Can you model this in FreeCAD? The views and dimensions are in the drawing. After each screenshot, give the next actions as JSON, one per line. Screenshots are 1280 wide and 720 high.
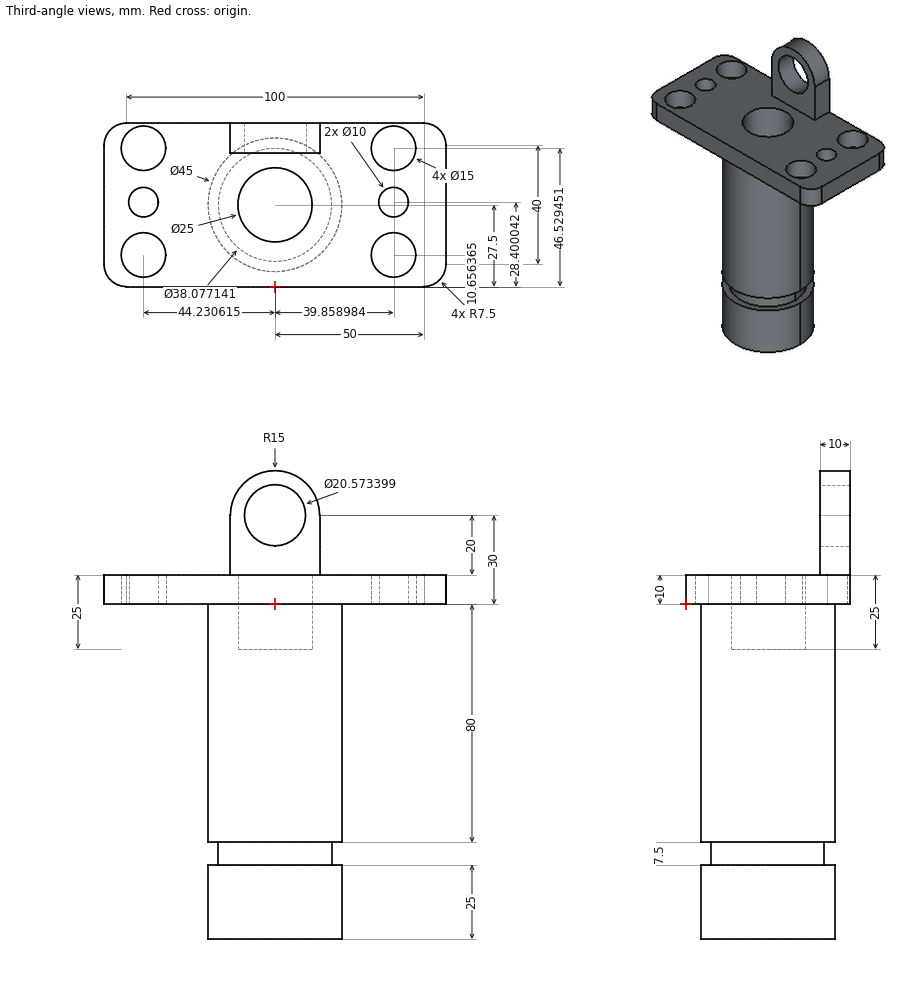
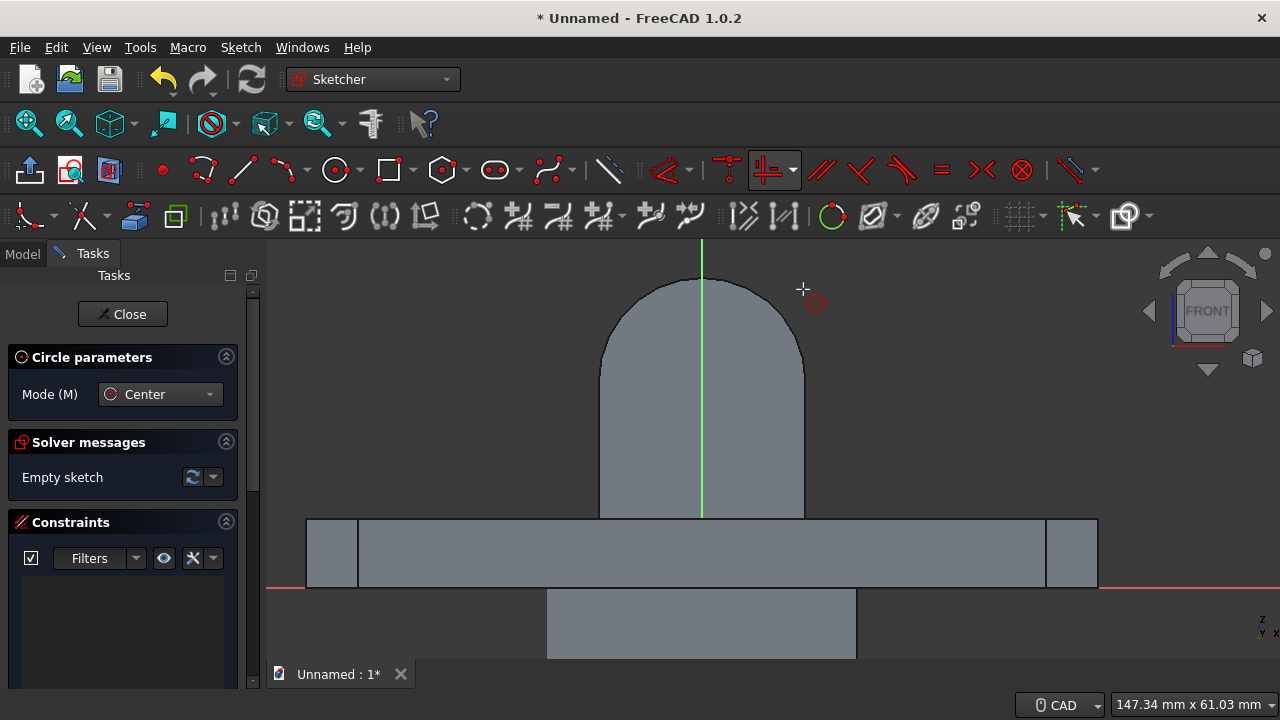
{"action": "left_click", "coordinate": [702, 381]}
{"action": "left_click", "coordinate": [752, 331]}
{"action": "key", "text": "Escape"}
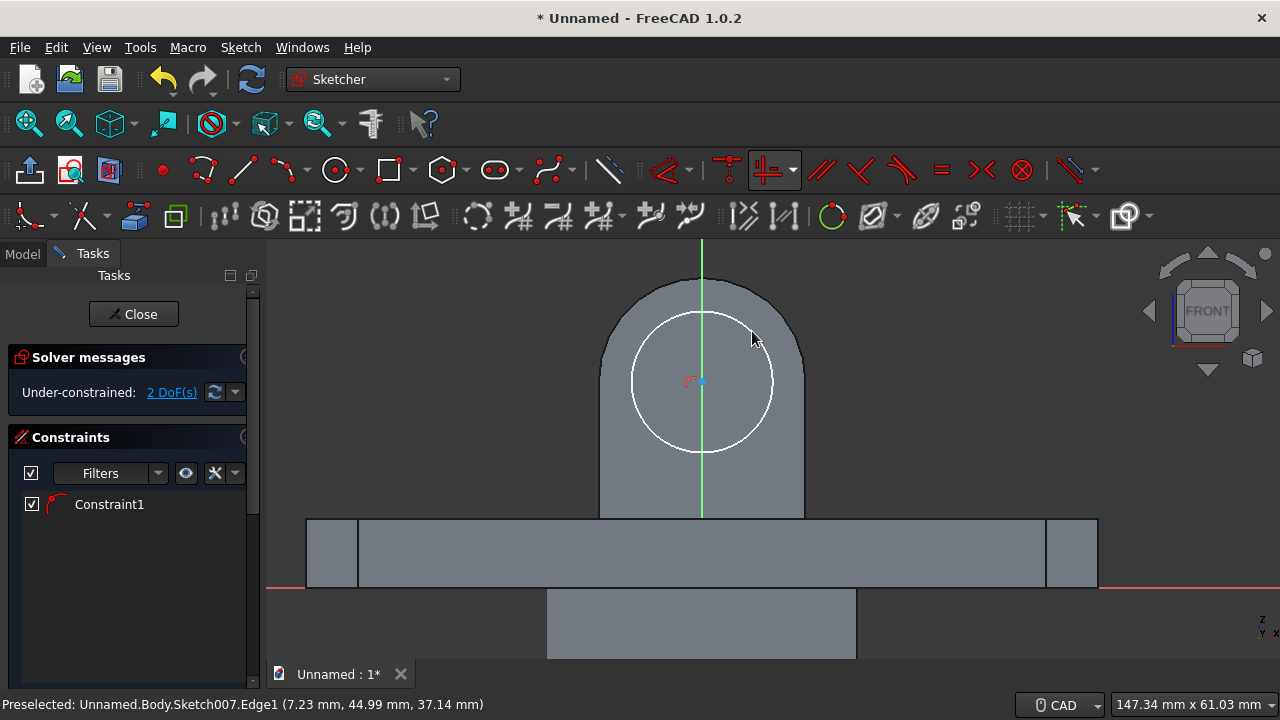
{"action": "left_click", "coordinate": [664, 170]}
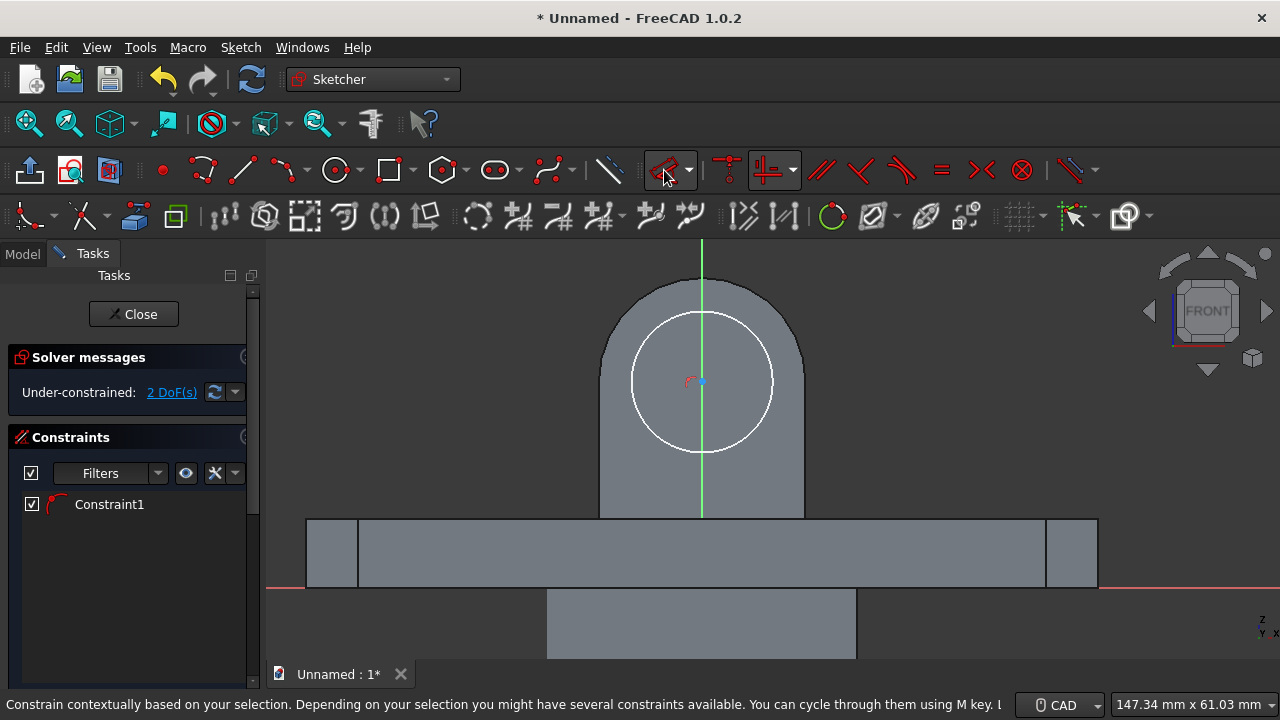
{"action": "left_click", "coordinate": [752, 332]}
{"action": "left_click", "coordinate": [775, 309]}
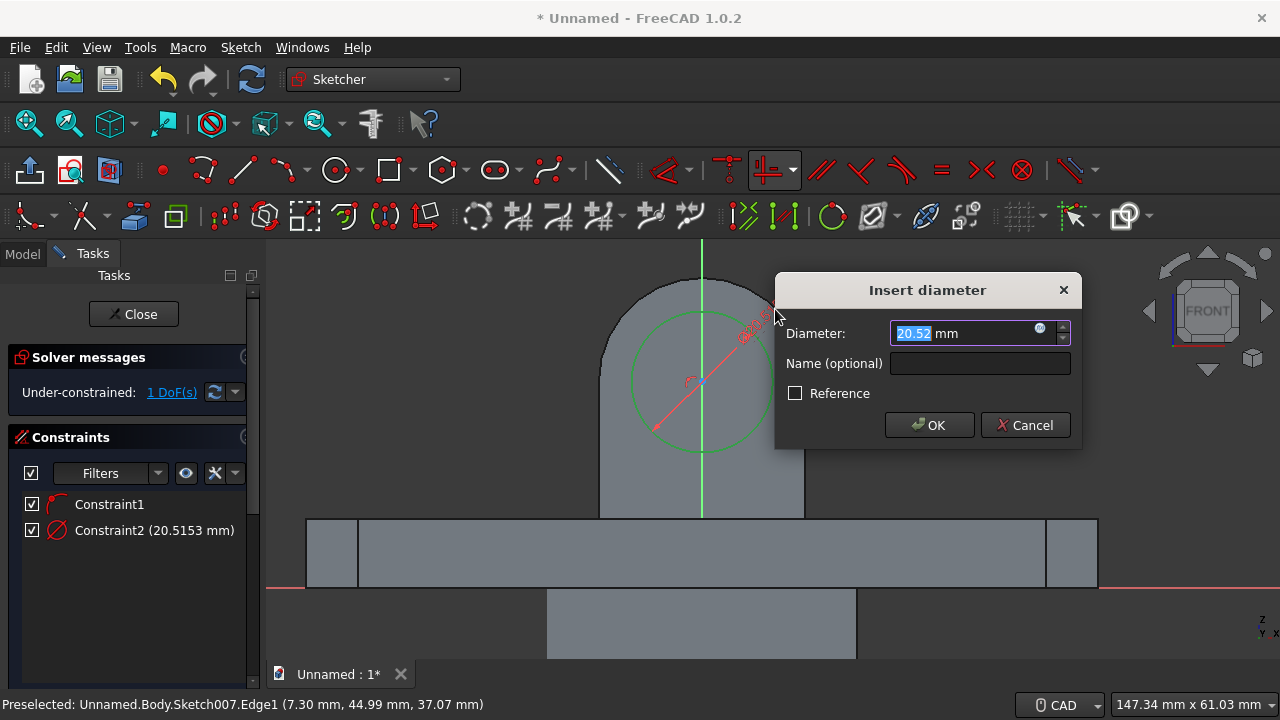
{"action": "type", "text": "20.573399"}
{"action": "key", "text": "Return"}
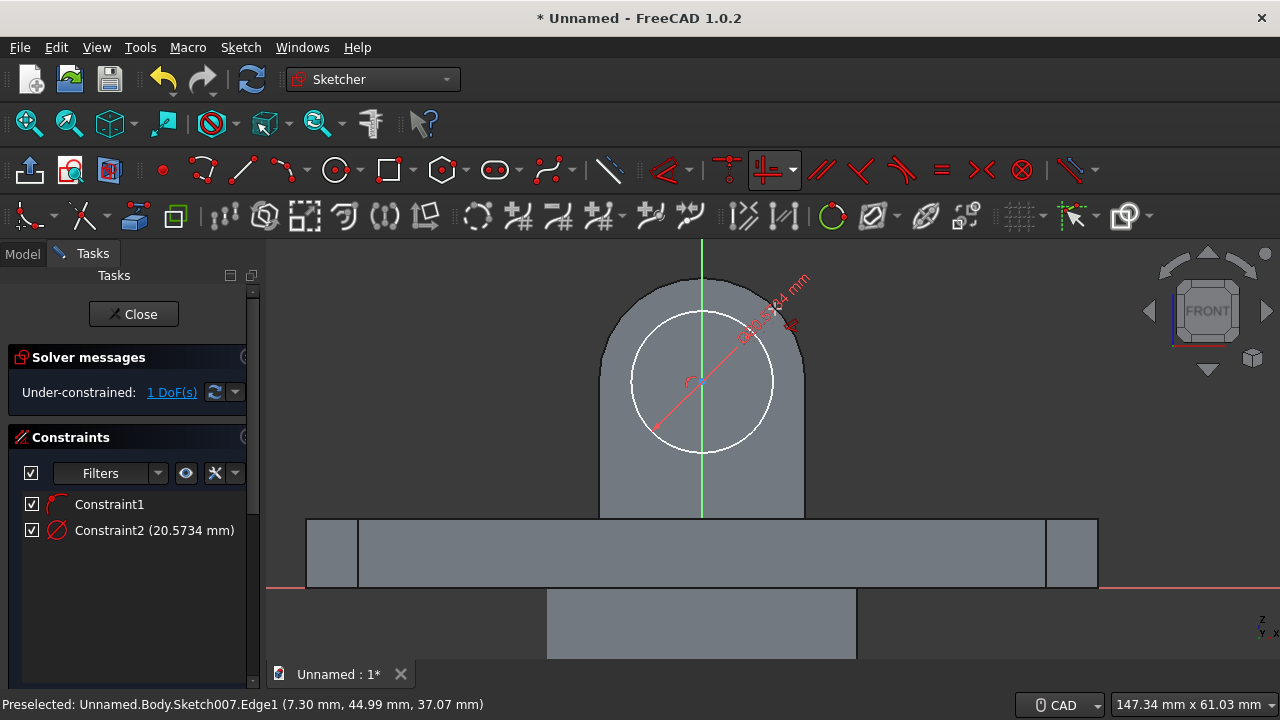
{"action": "left_click", "coordinate": [702, 382]}
{"action": "left_click", "coordinate": [736, 485]}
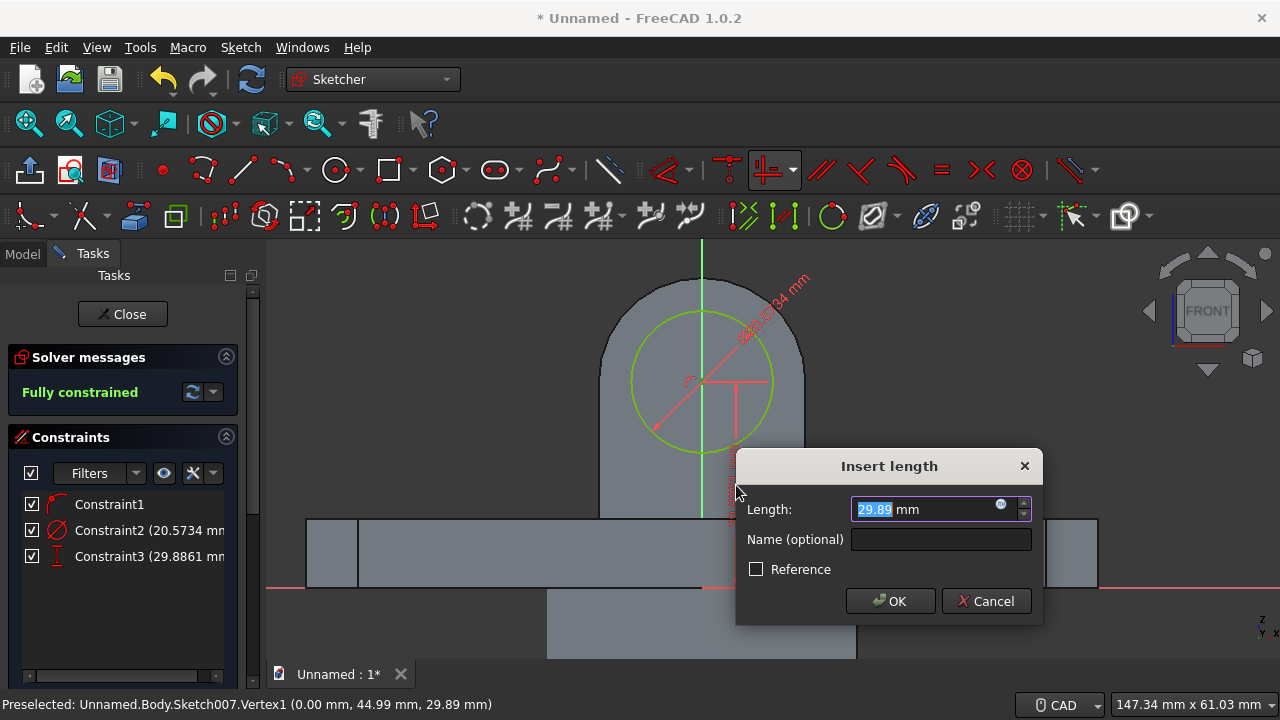
{"action": "type", "text": "30"}
{"action": "key", "text": "Return"}
{"action": "key", "text": "Escape"}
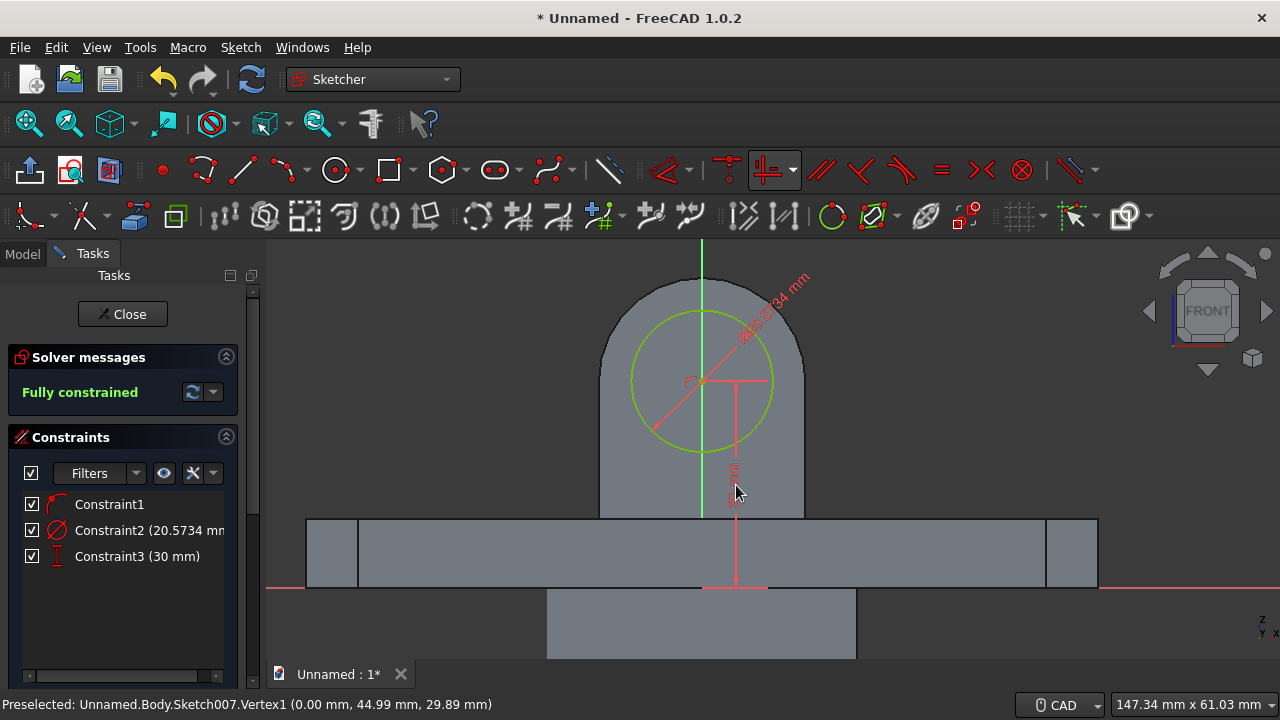
{"action": "left_click", "coordinate": [123, 314]}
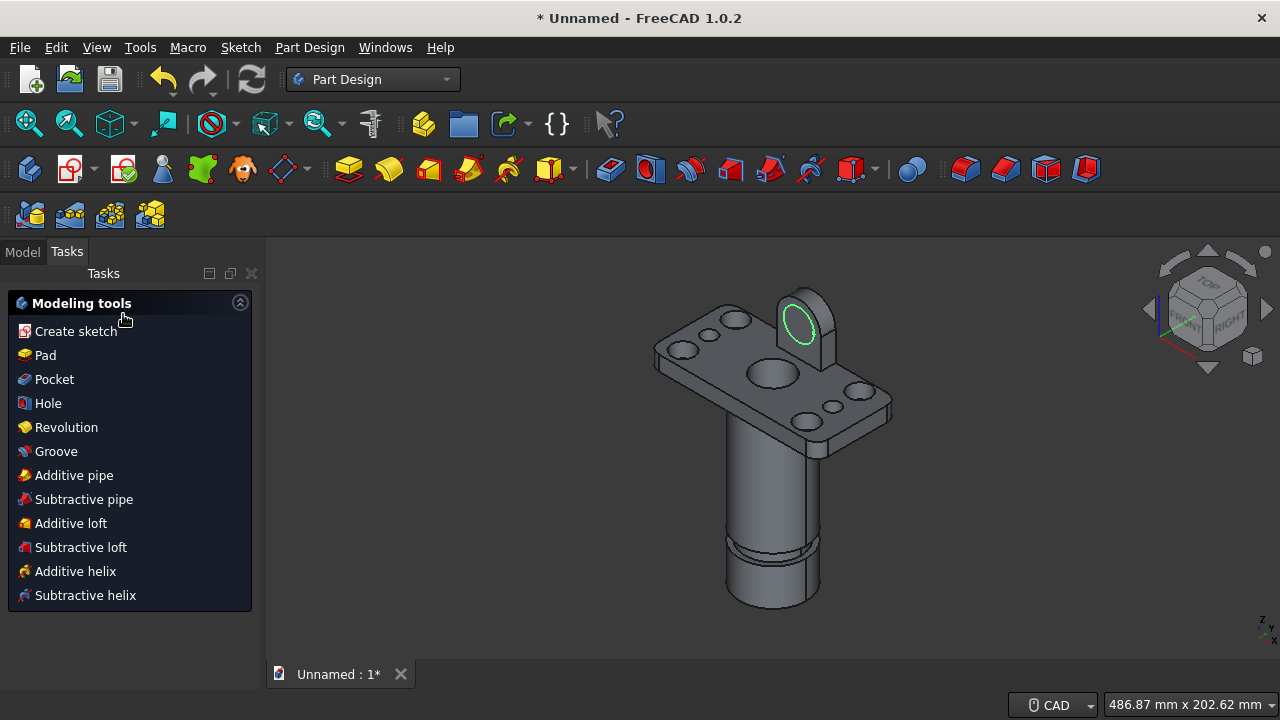
{"action": "left_click", "coordinate": [612, 170]}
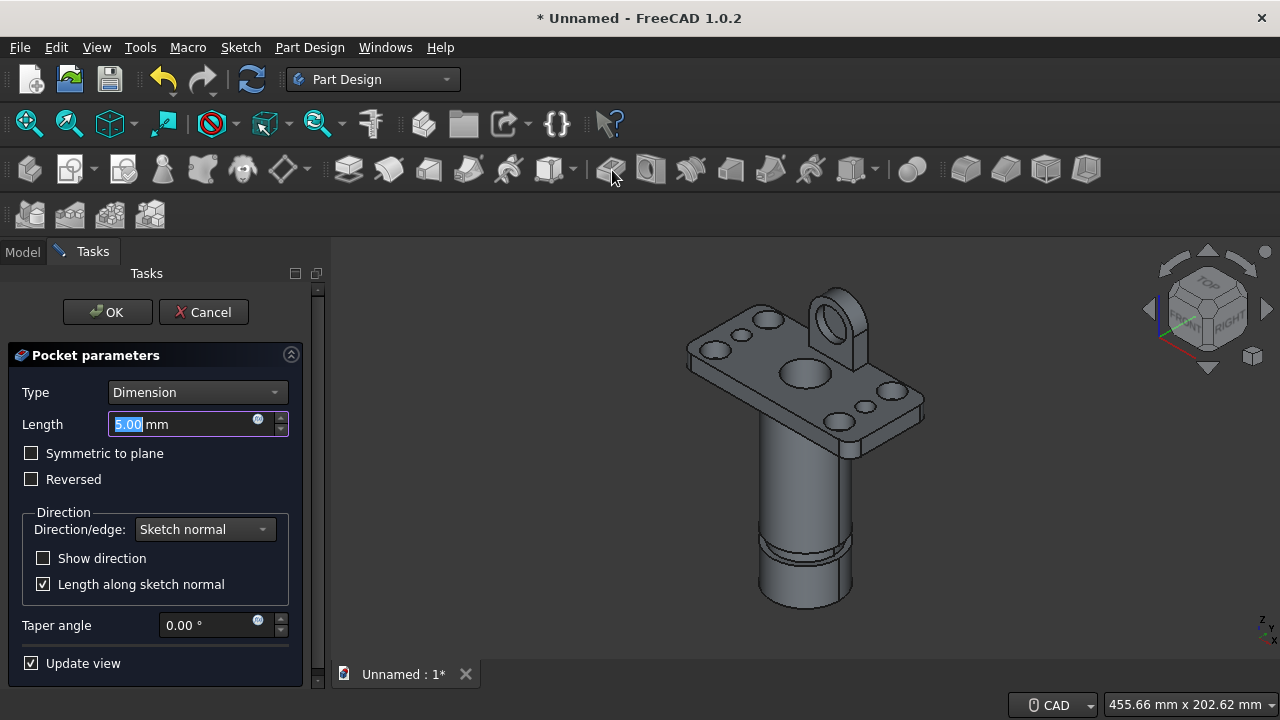
{"action": "type", "text": "10"}
{"action": "key", "text": "Tab"}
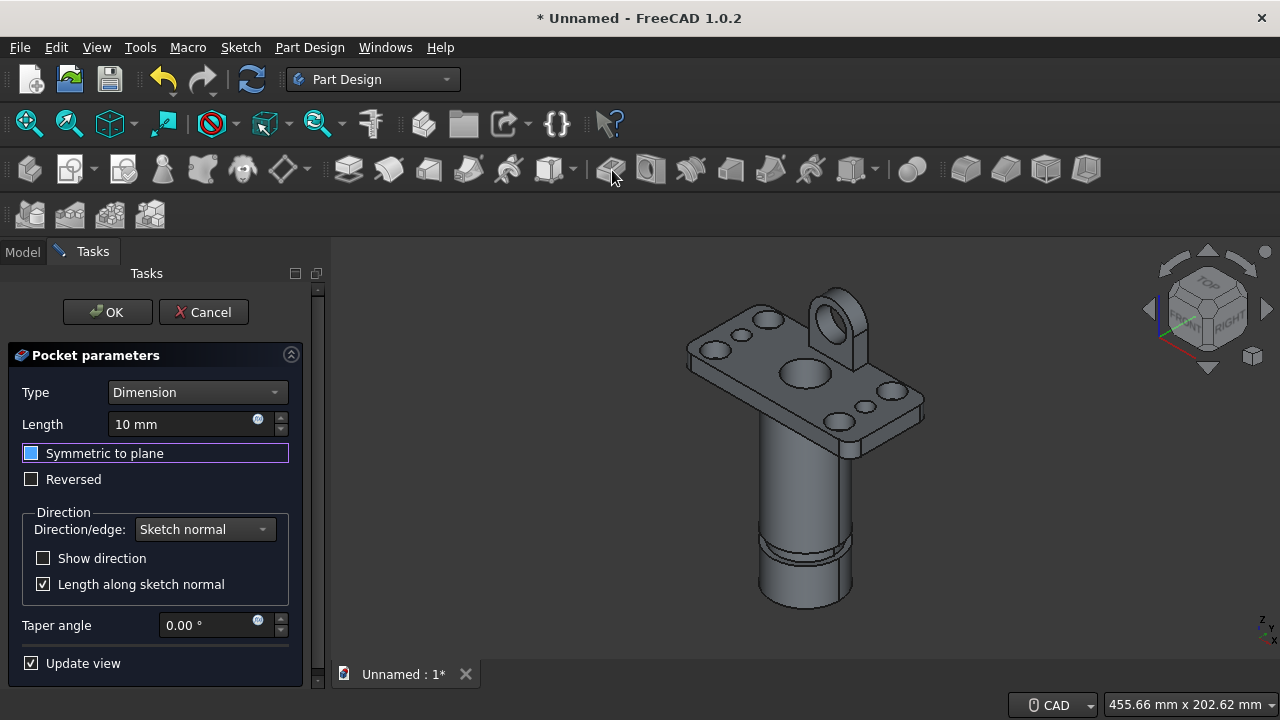
{"action": "left_click", "coordinate": [108, 312]}